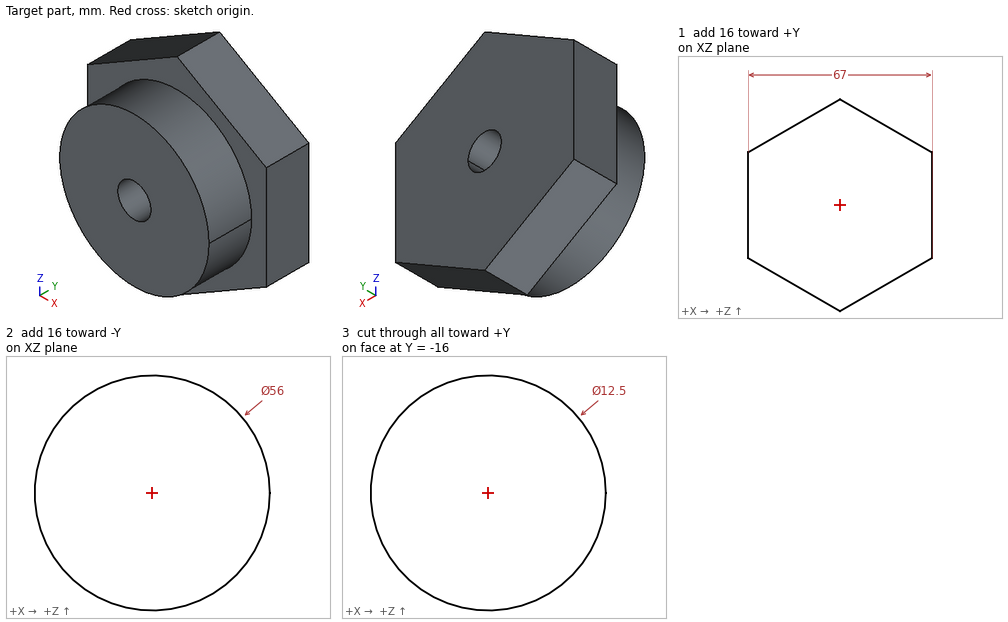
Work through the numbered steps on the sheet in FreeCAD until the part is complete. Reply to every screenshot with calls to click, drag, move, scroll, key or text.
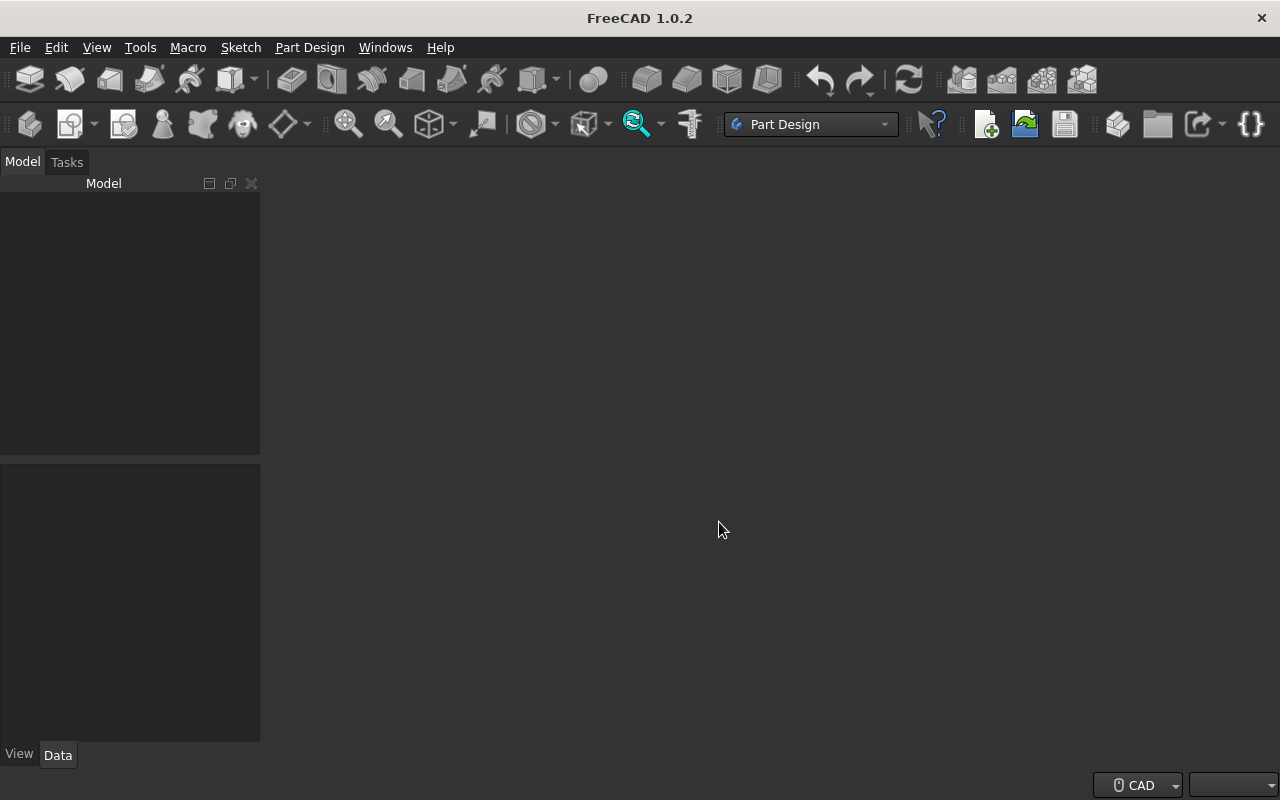
click(986, 124)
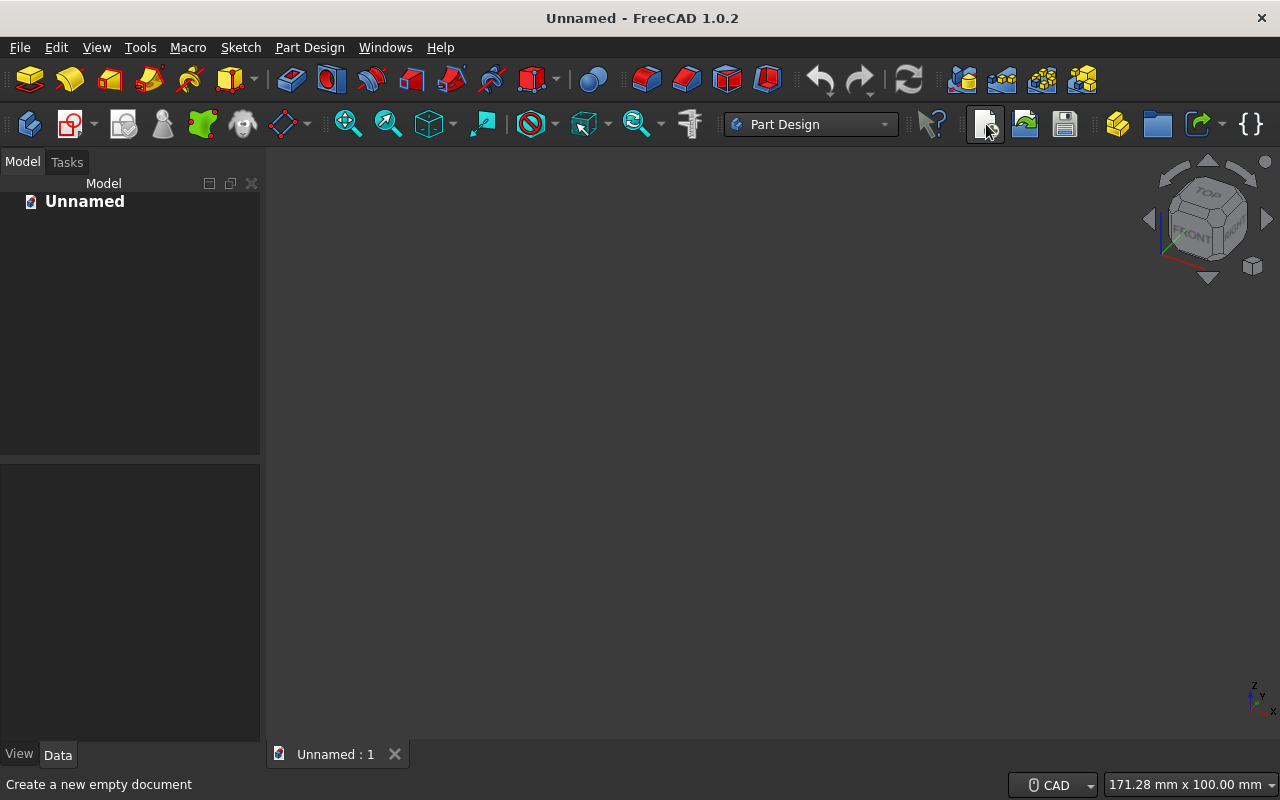
click(70, 124)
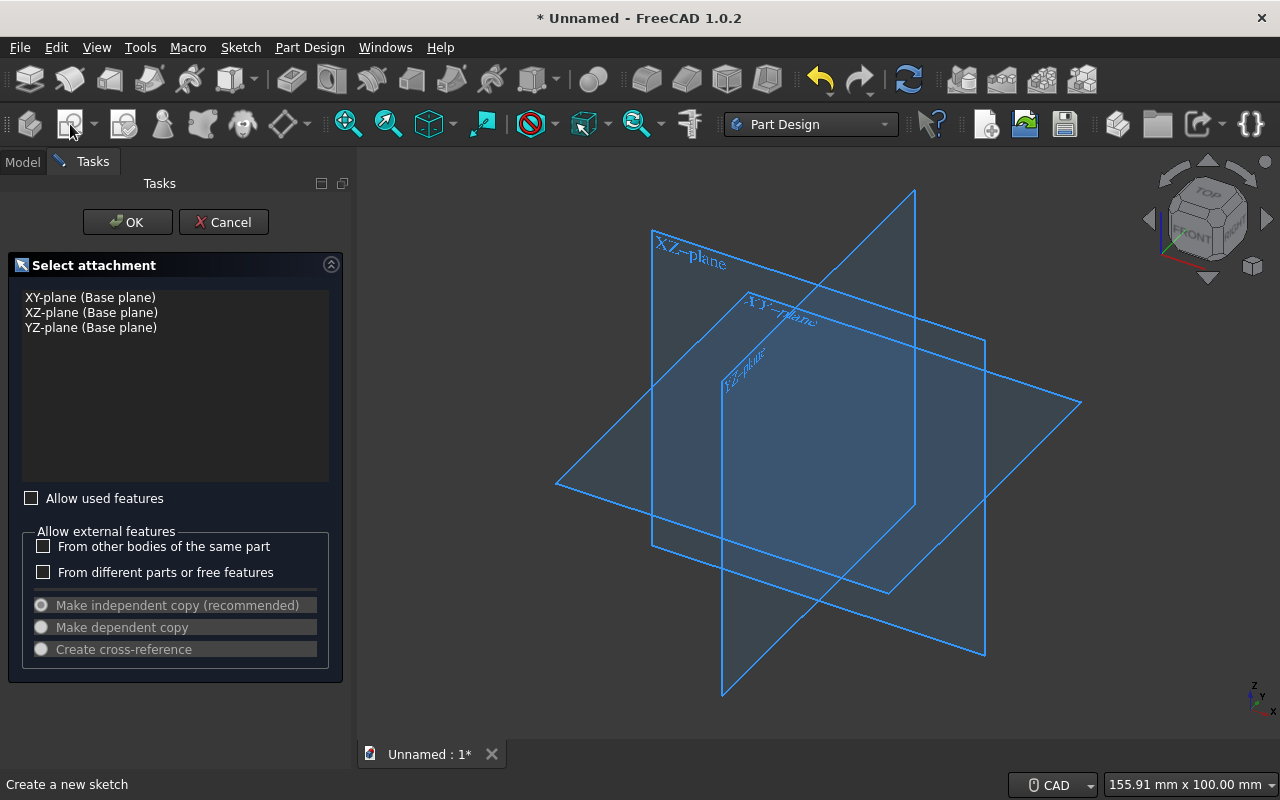
click(82, 312)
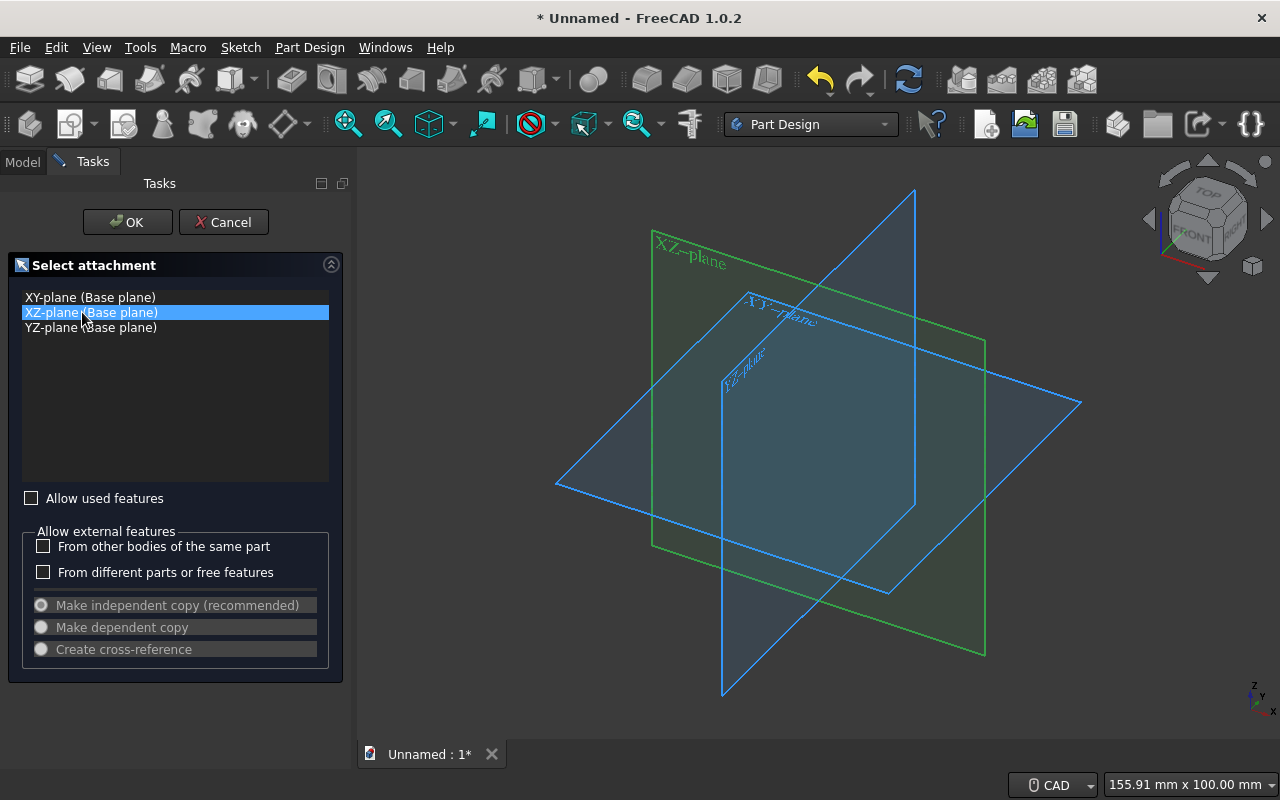
click(128, 222)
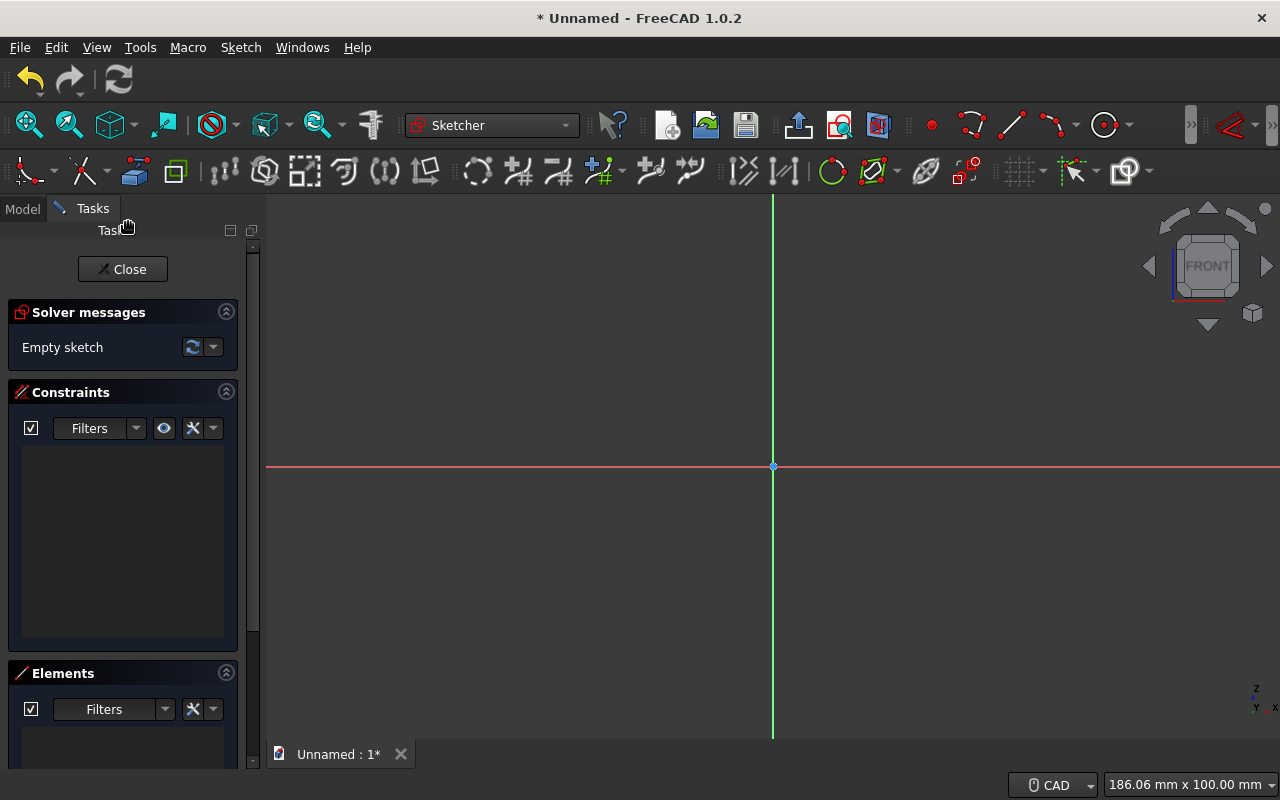
key(g)
key(p)
key(6)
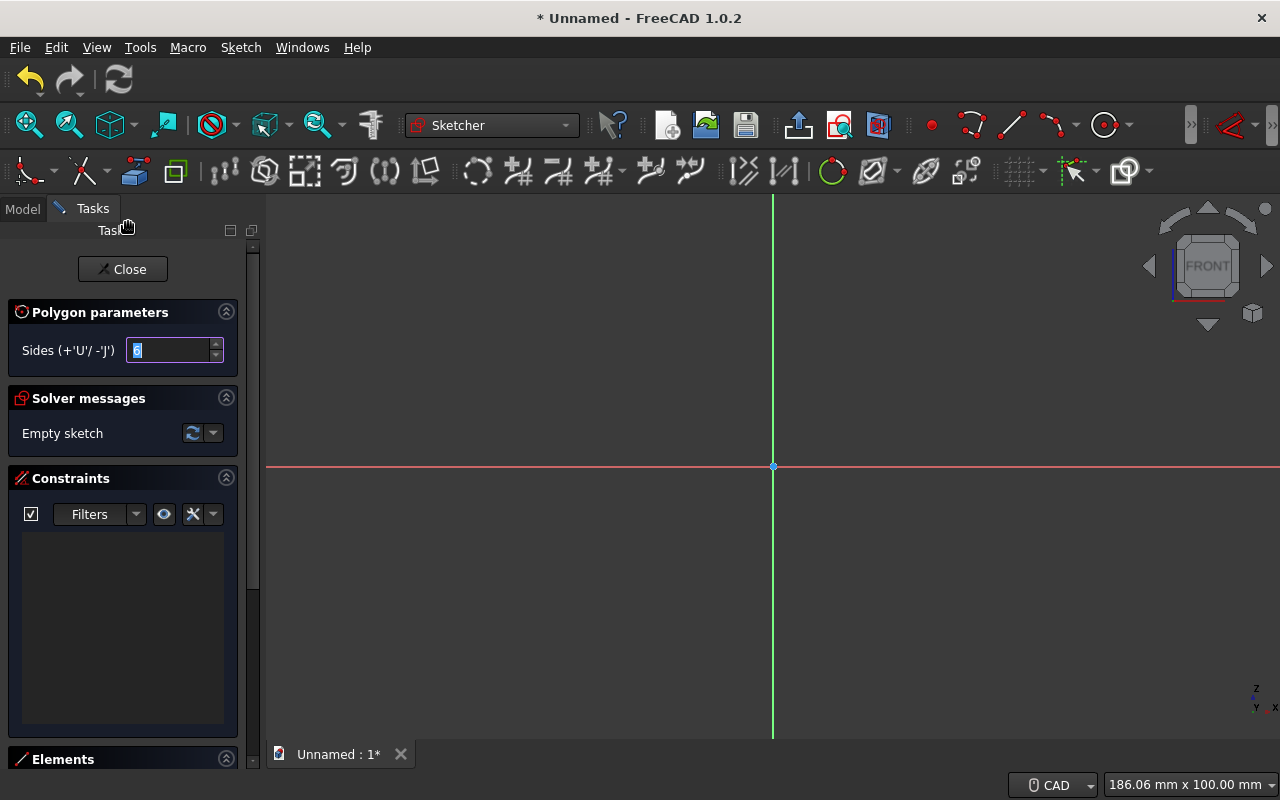
click(773, 466)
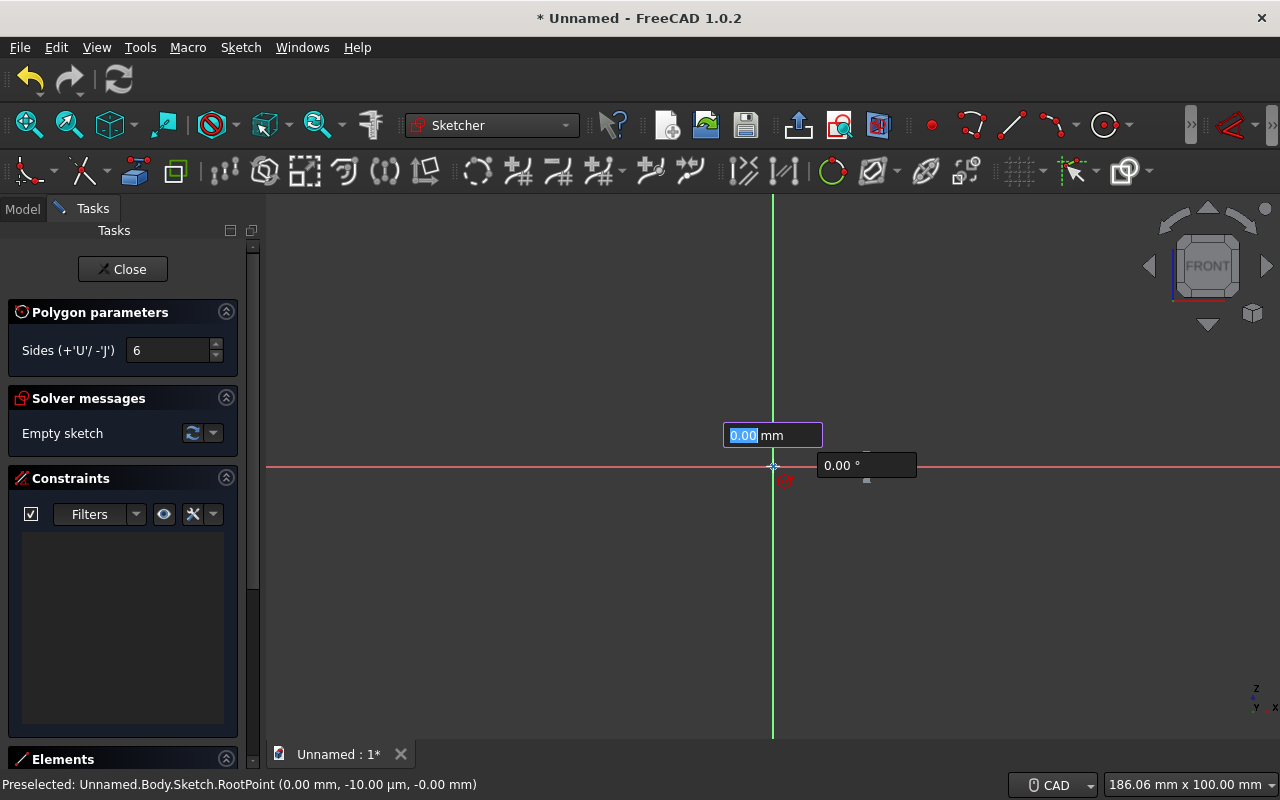
click(773, 256)
right_click(773, 256)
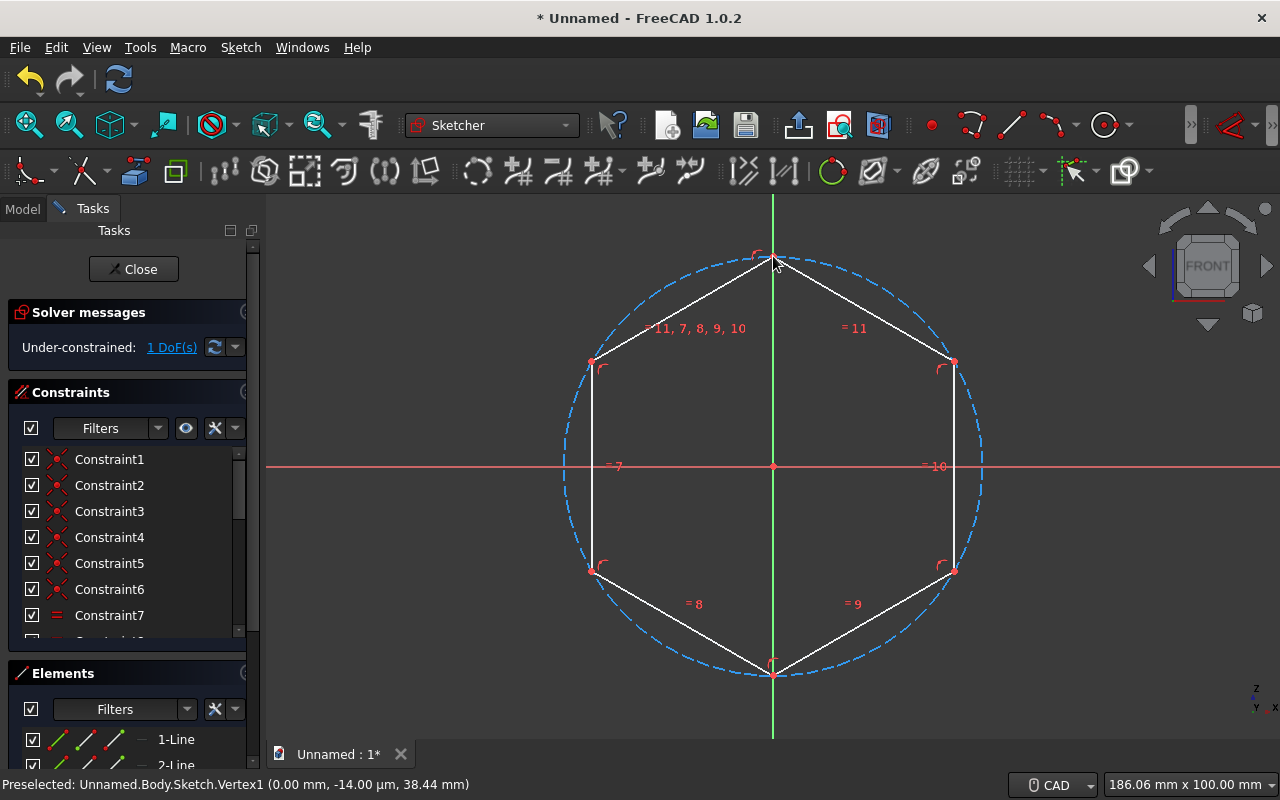
key(d)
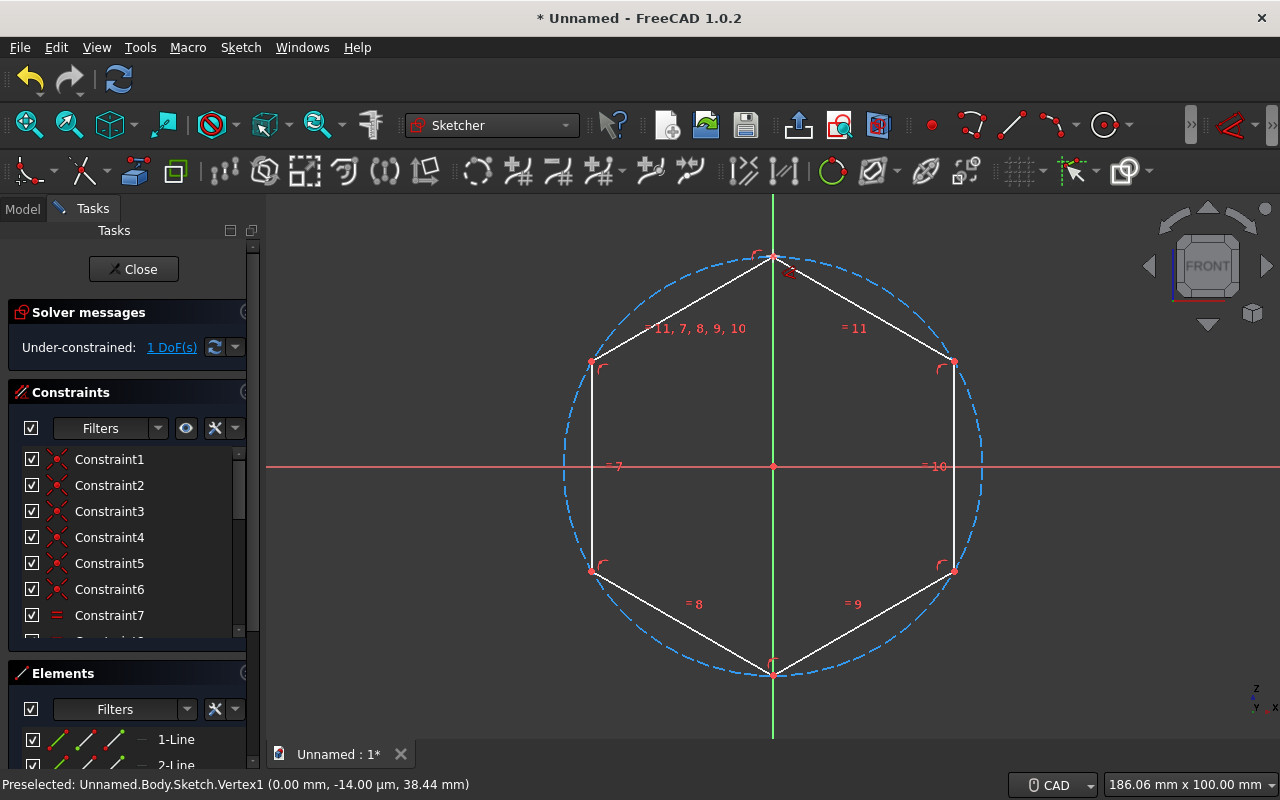
click(592, 362)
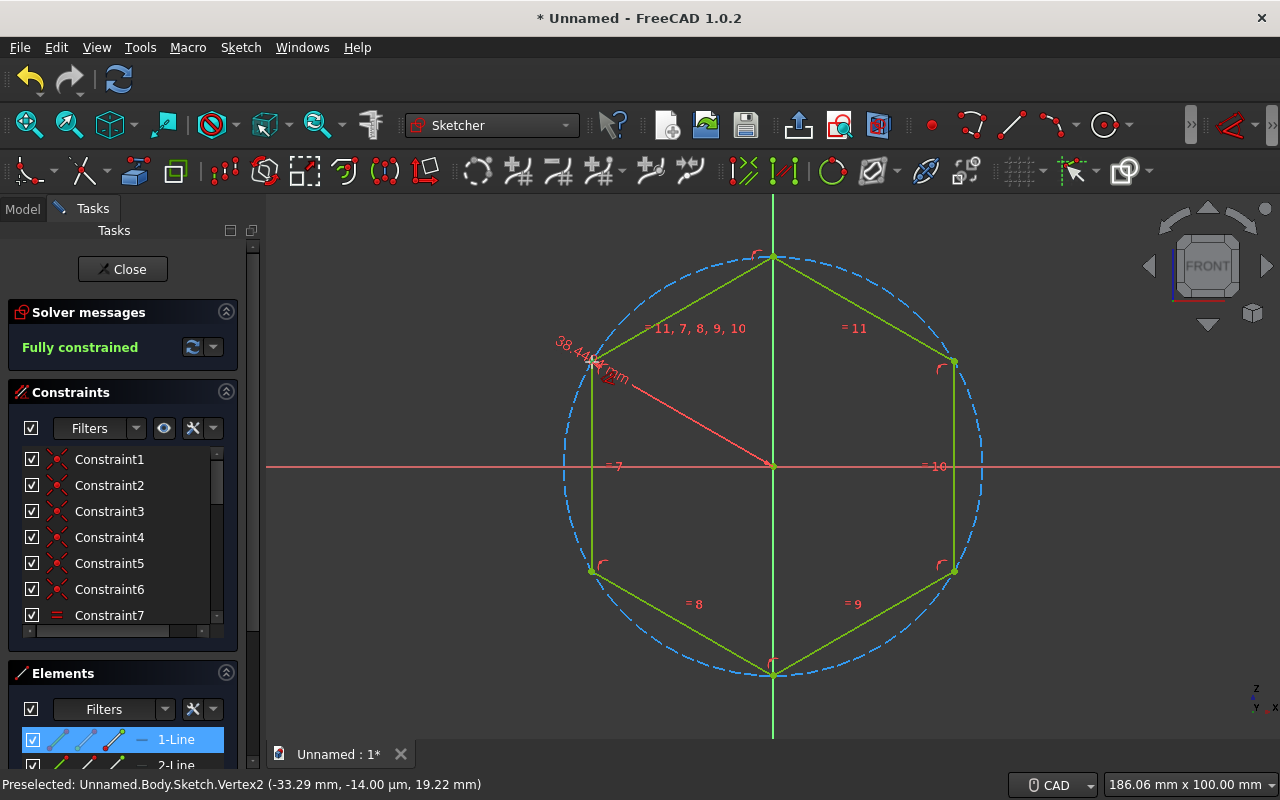
click(954, 571)
click(690, 605)